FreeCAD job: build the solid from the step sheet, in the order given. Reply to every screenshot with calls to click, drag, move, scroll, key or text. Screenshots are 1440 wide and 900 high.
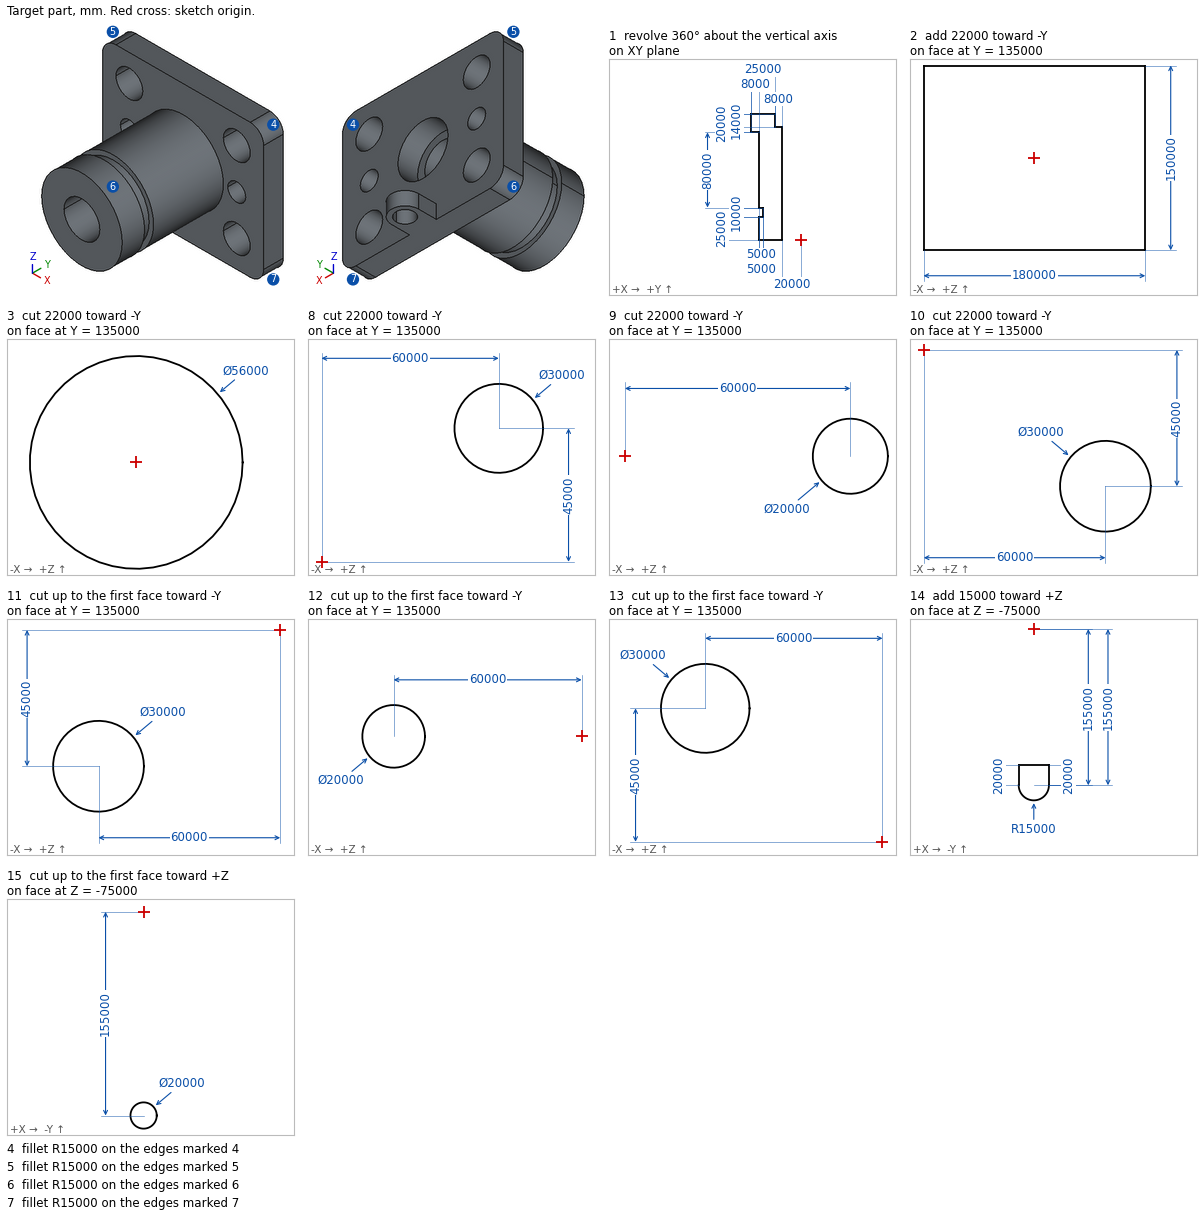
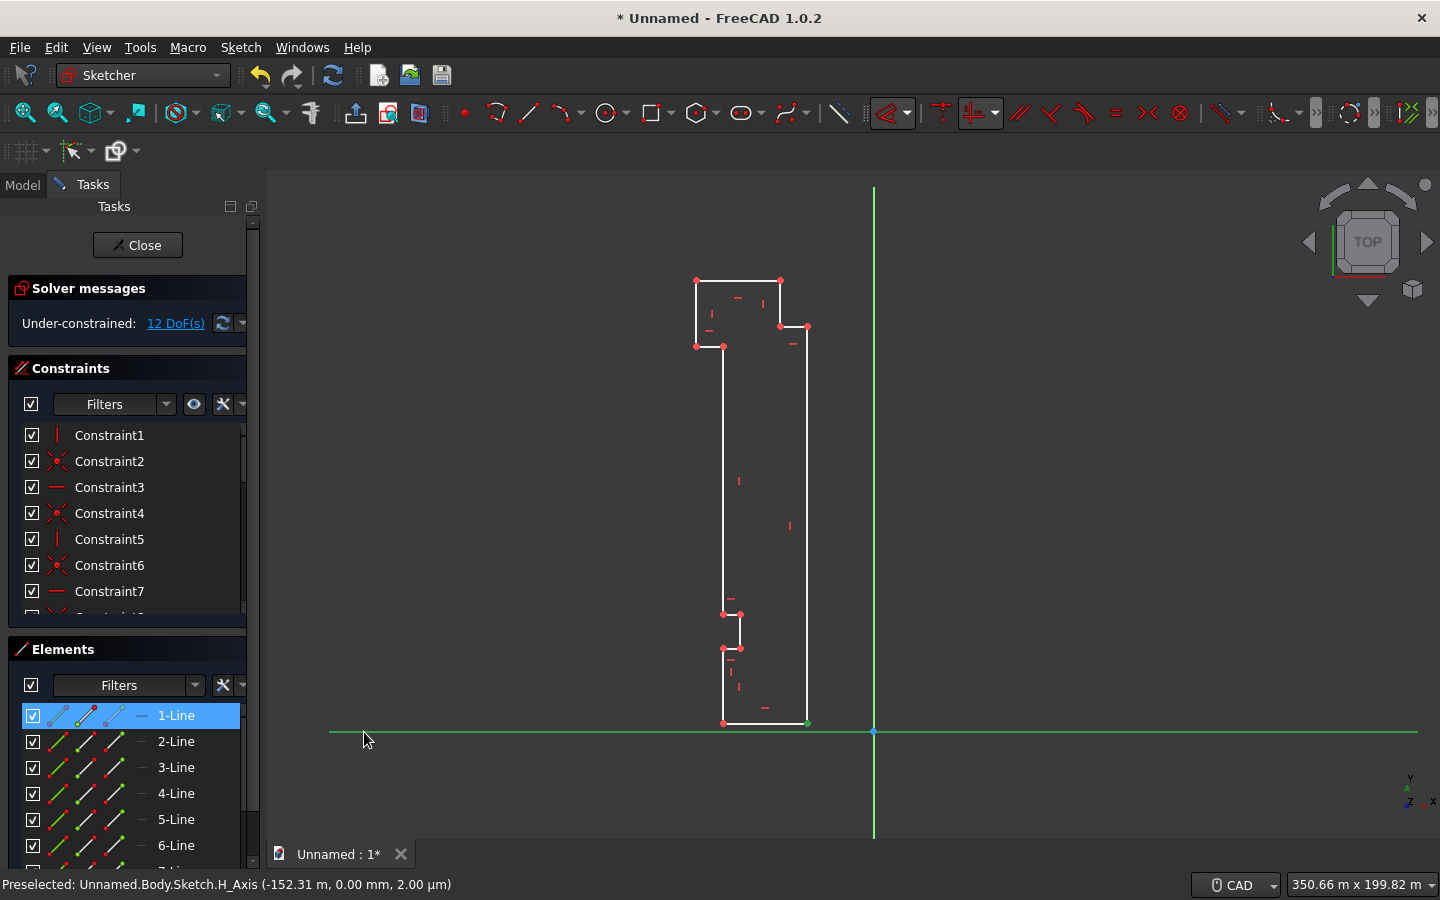
click(942, 114)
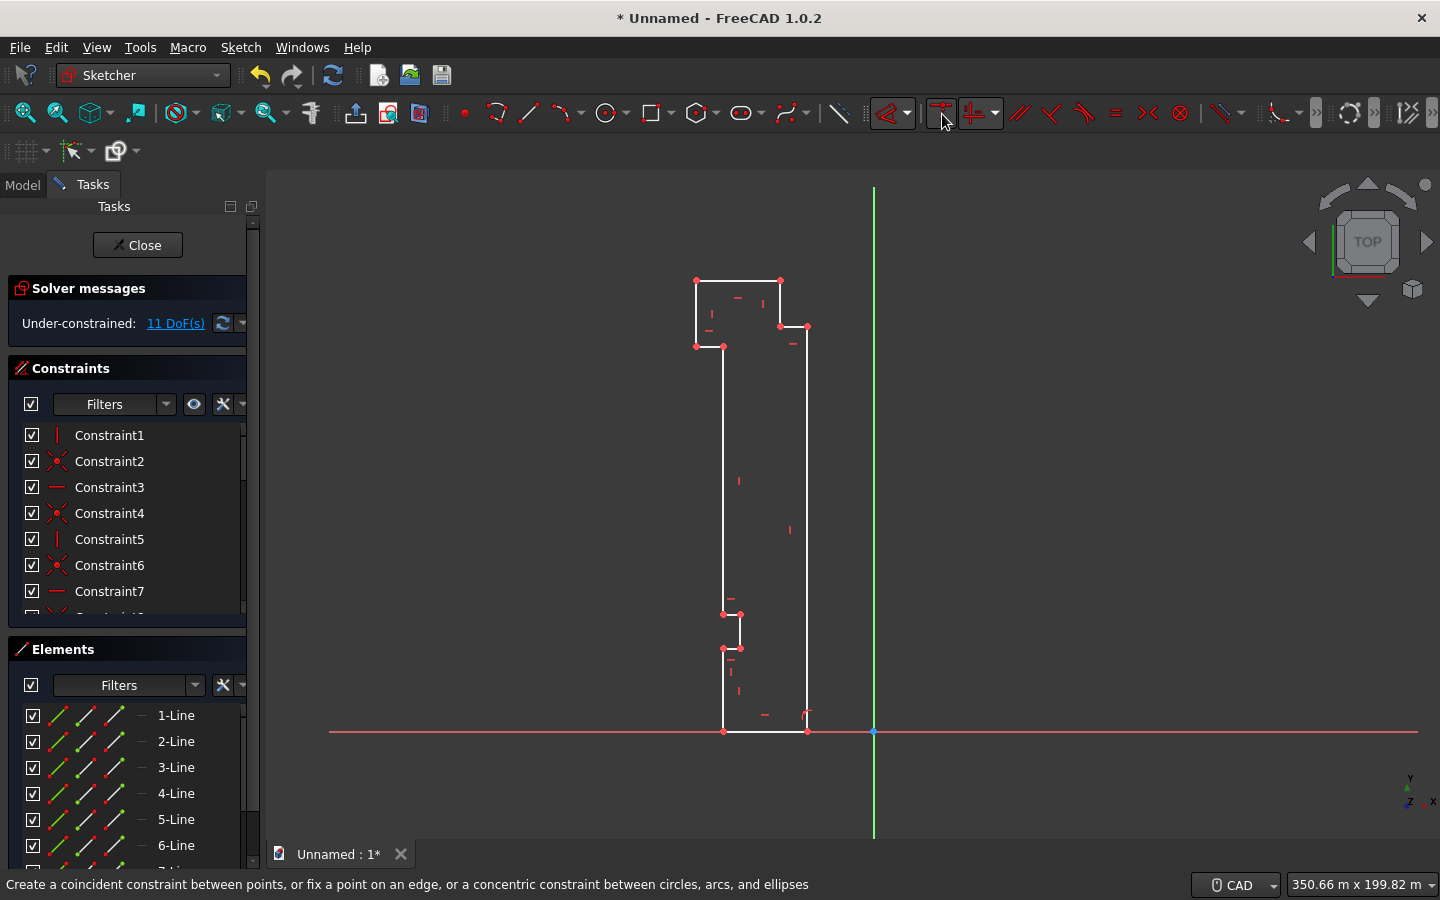
click(886, 114)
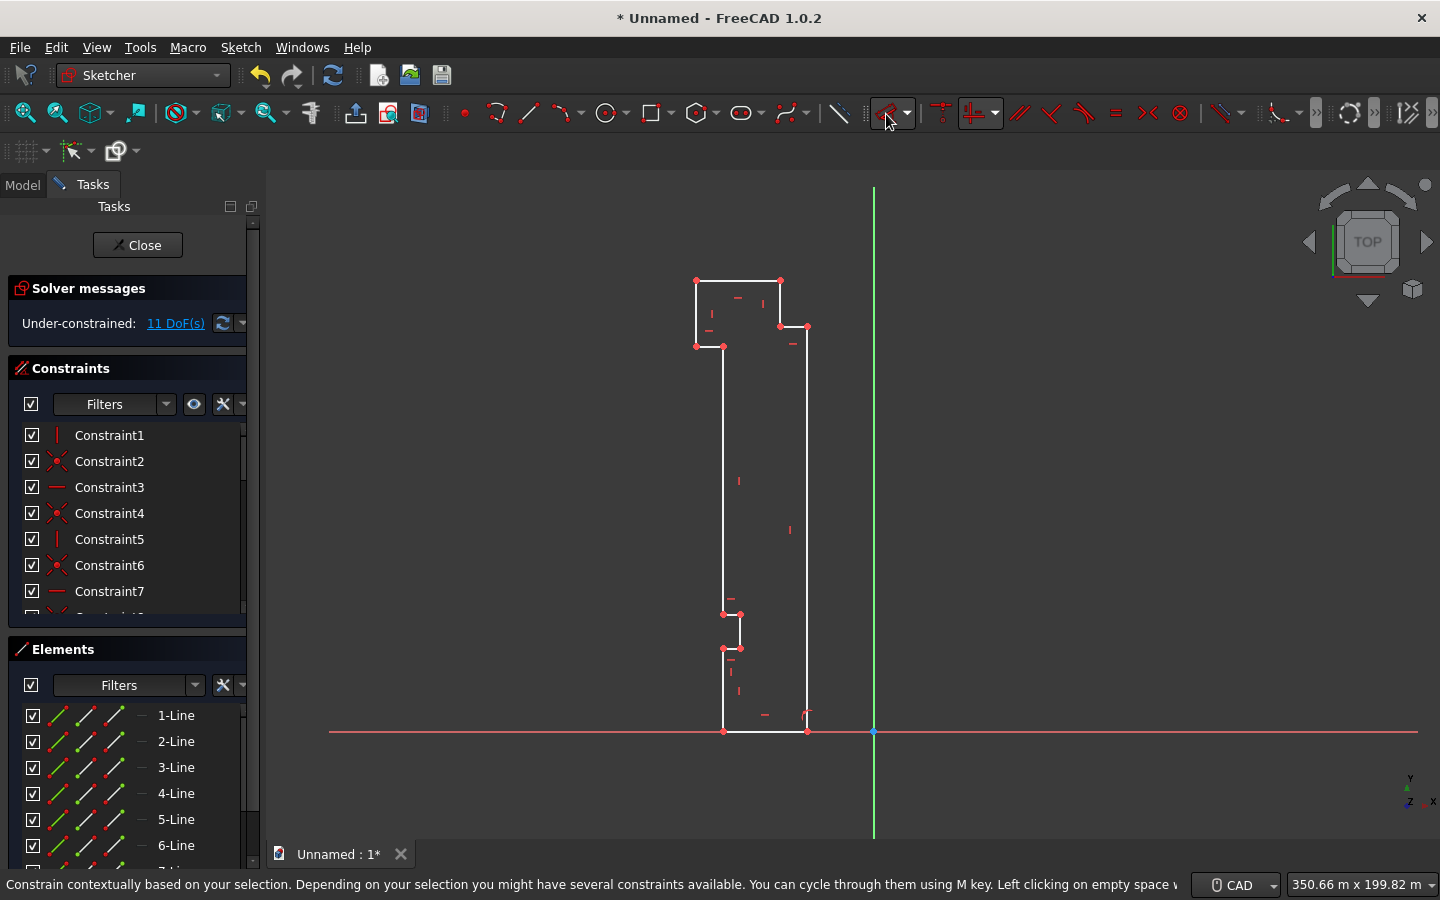
scroll(796, 327, up, 2)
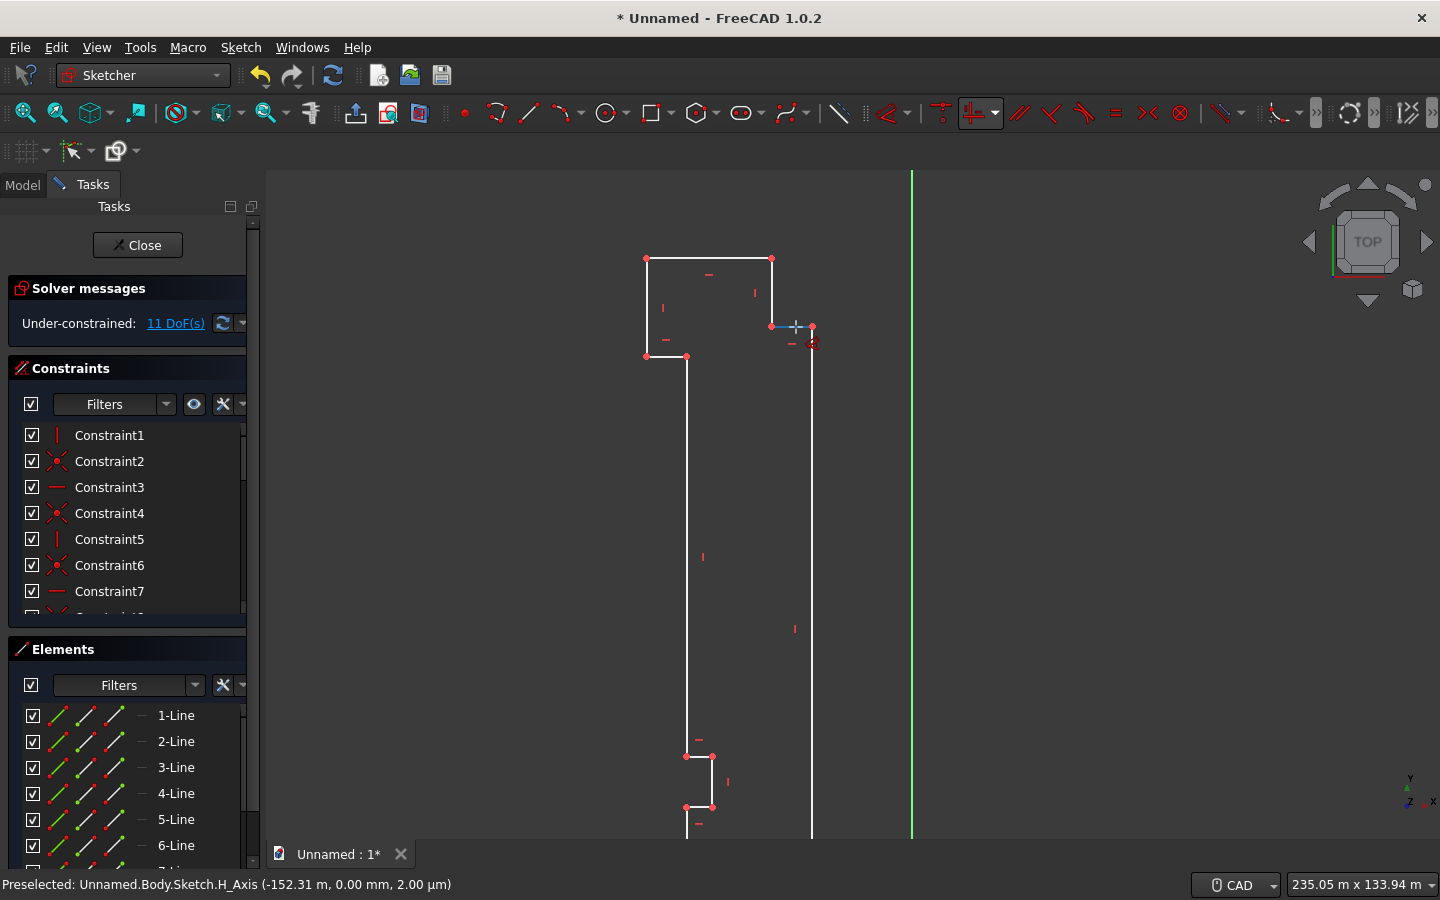
click(796, 327)
click(792, 293)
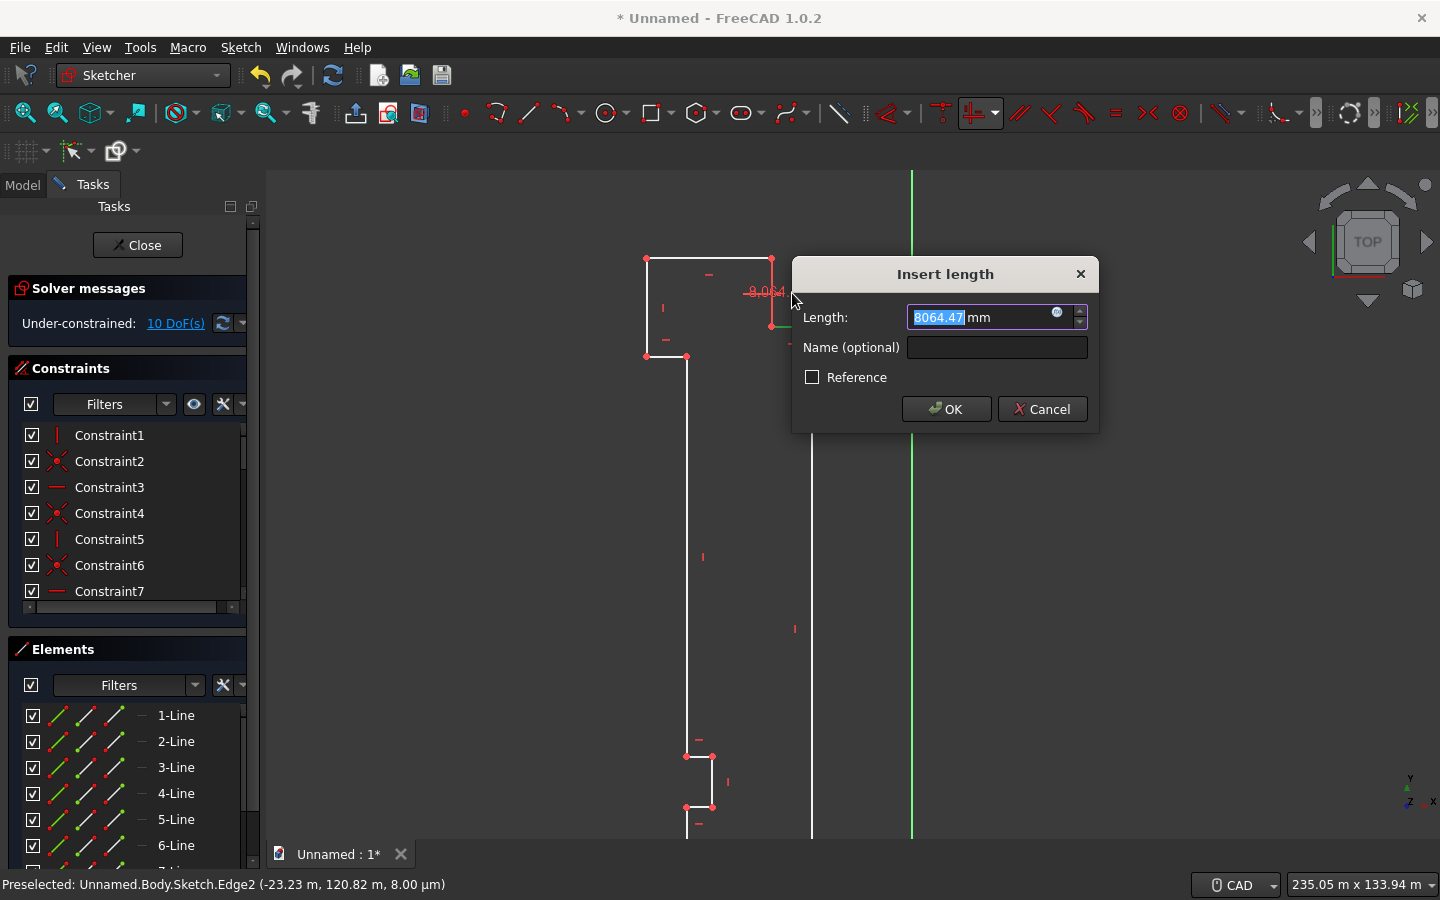
text(8000)
key(Return)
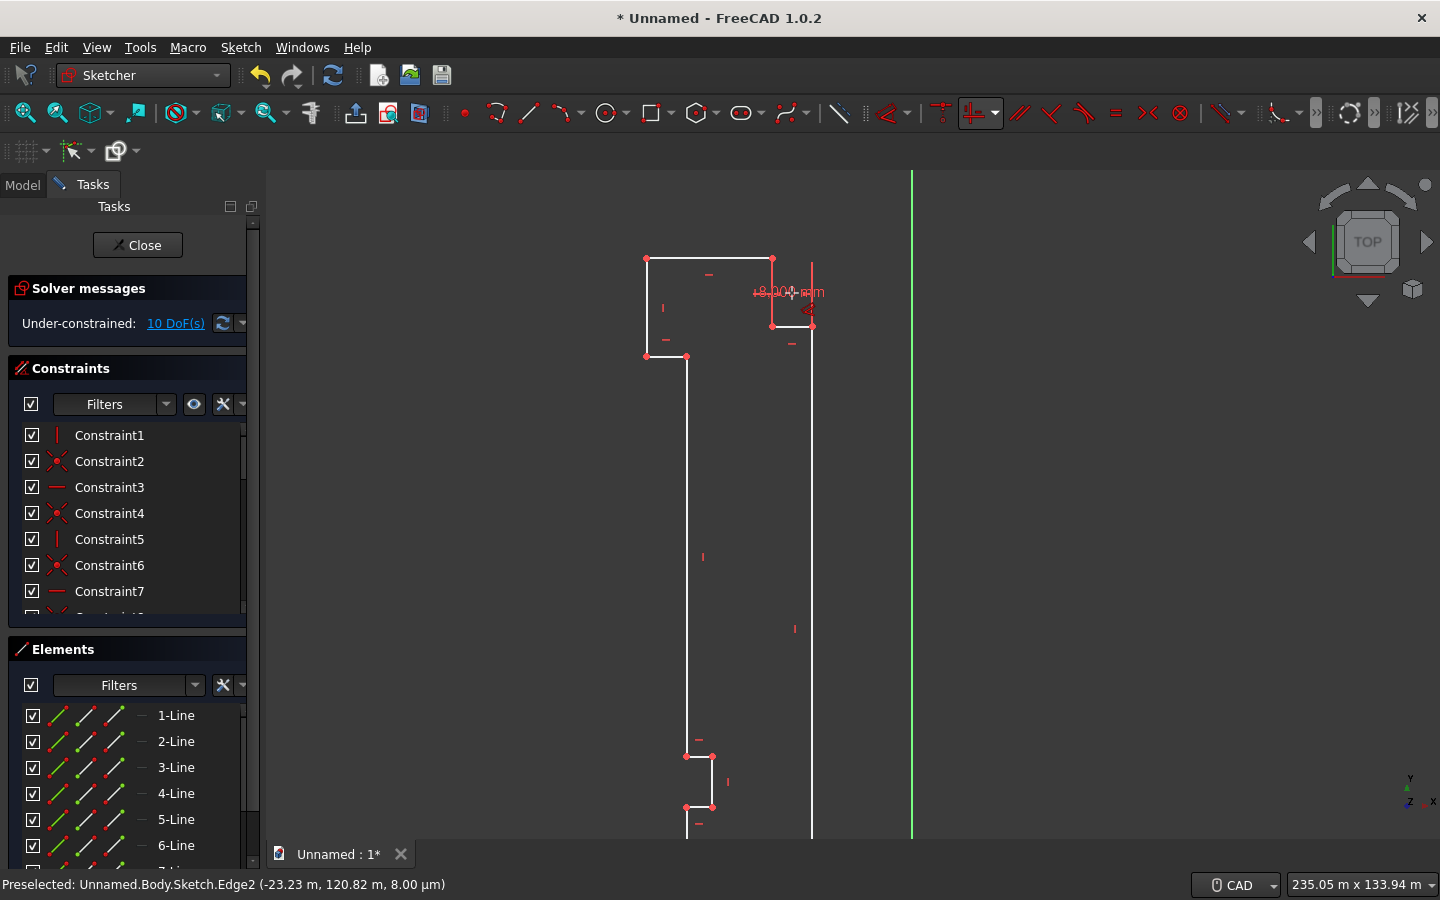
click(659, 357)
click(667, 323)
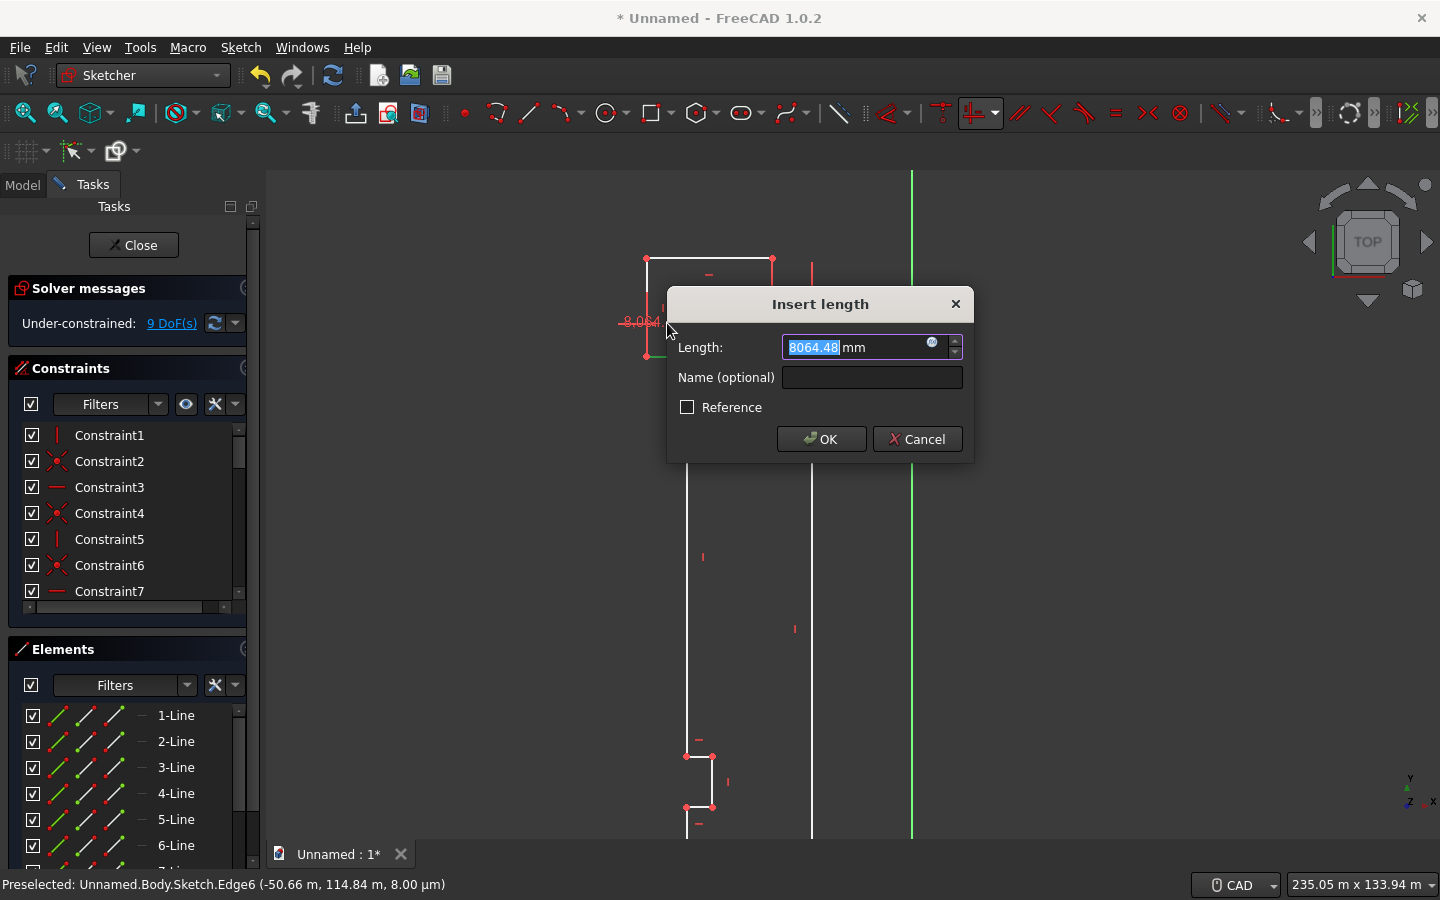
text(8000)
key(Return)